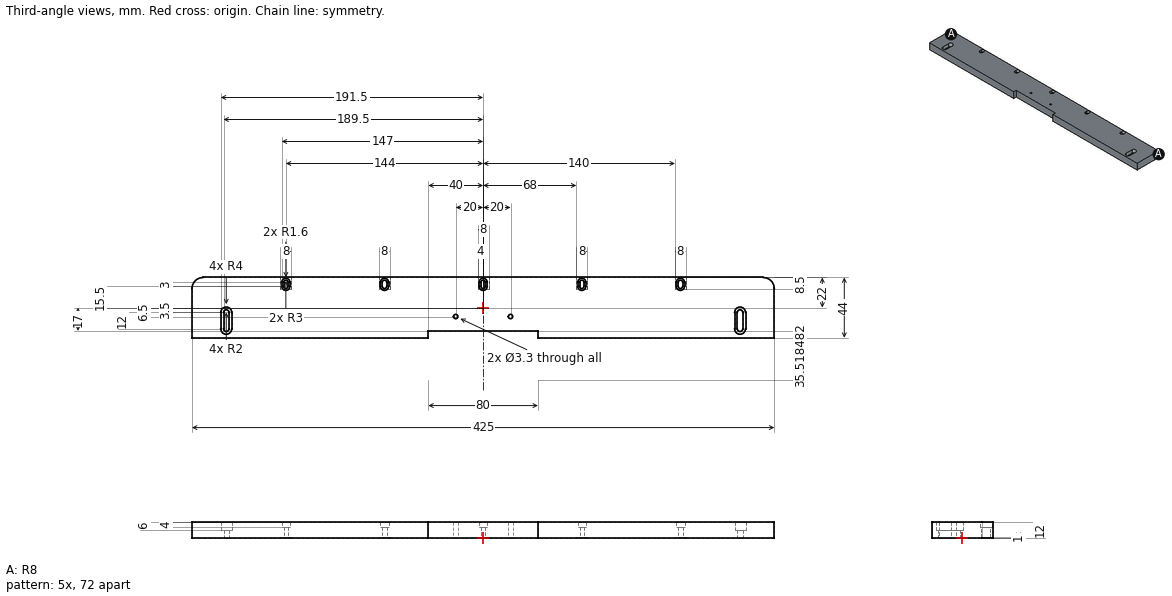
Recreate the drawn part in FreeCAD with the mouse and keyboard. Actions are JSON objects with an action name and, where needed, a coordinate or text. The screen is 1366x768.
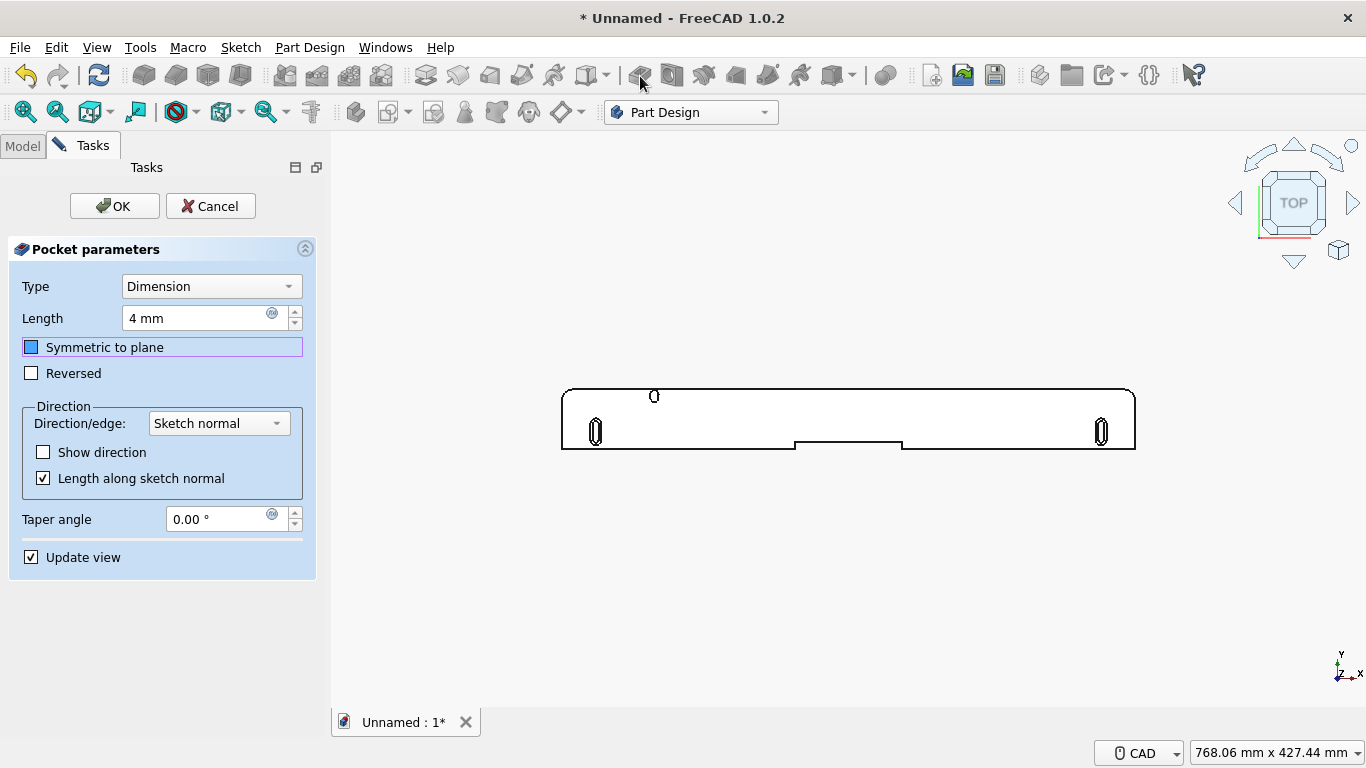
{"action": "left_click", "coordinate": [115, 206]}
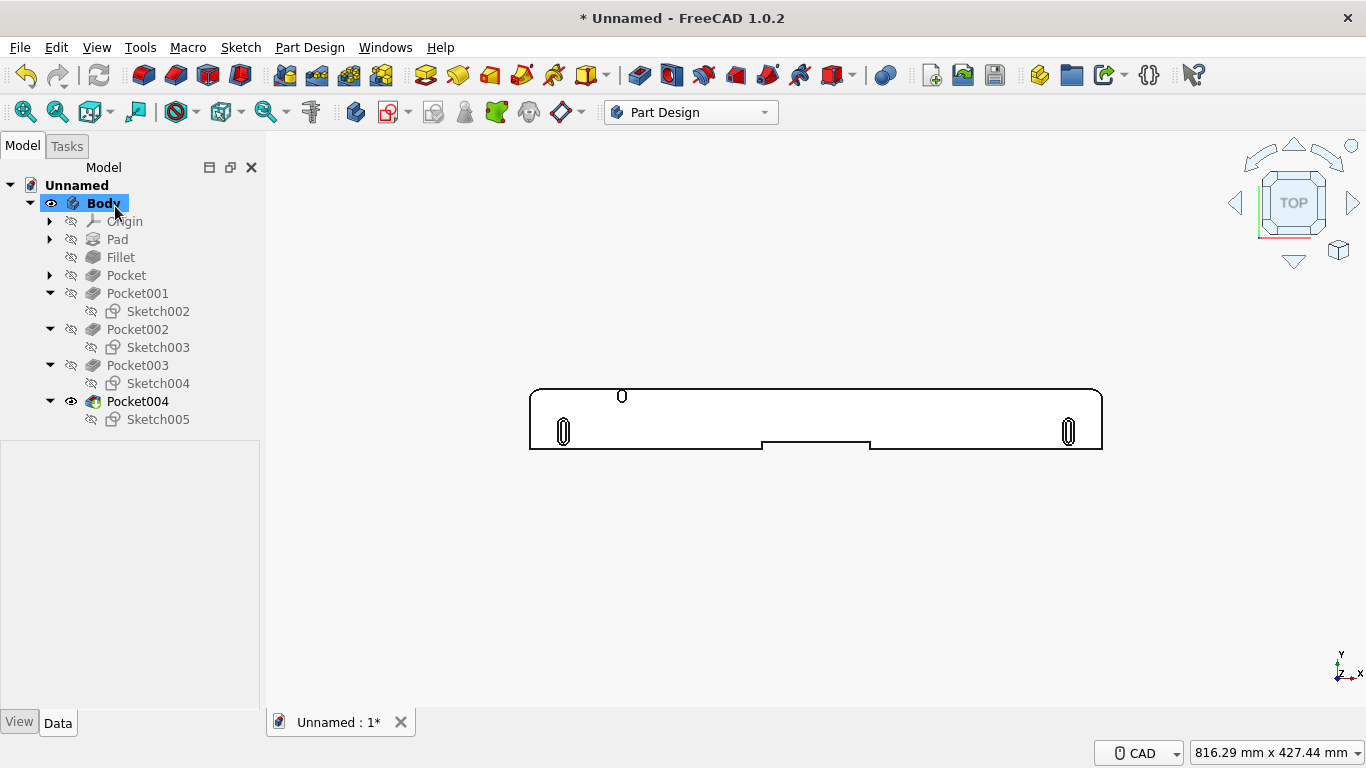
{"action": "scroll", "coordinate": [622, 393], "scroll_direction": "up", "scroll_amount": 6}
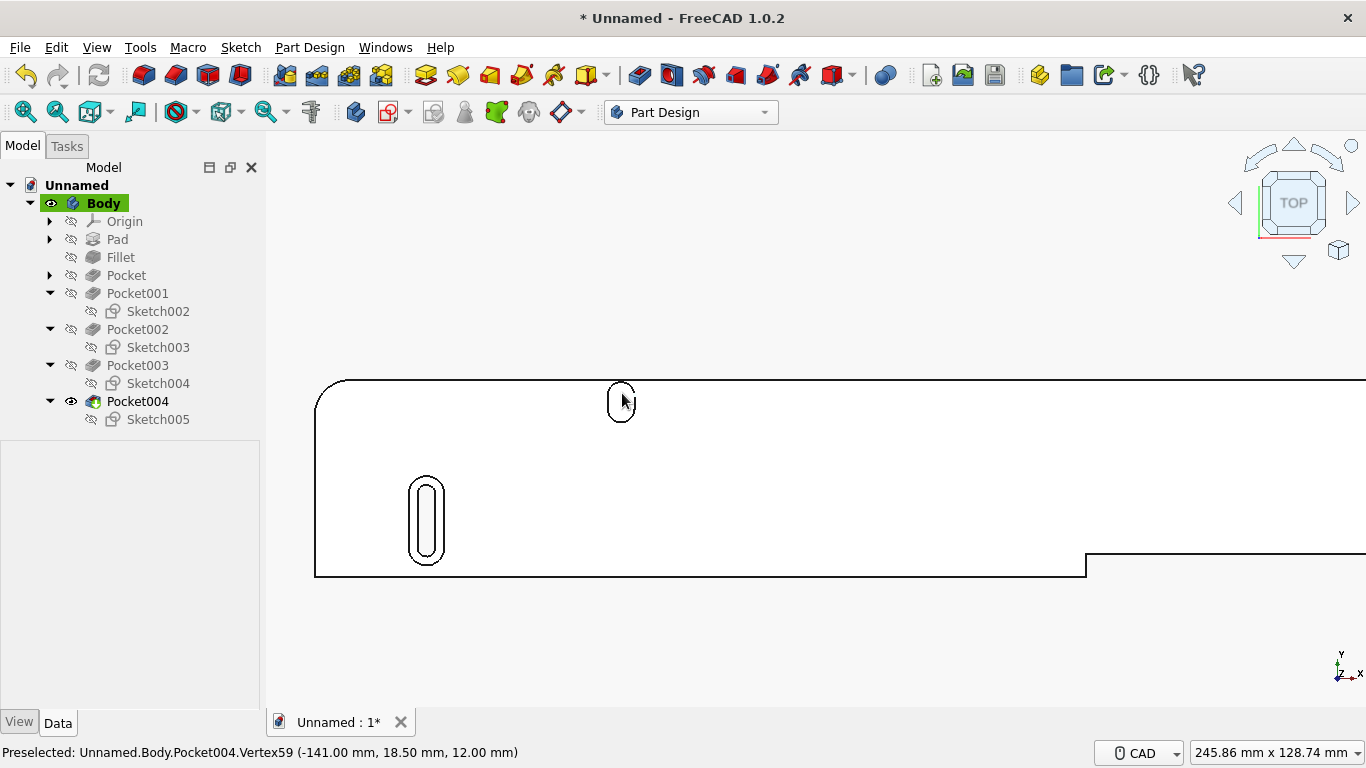
{"action": "left_click", "coordinate": [621, 395]}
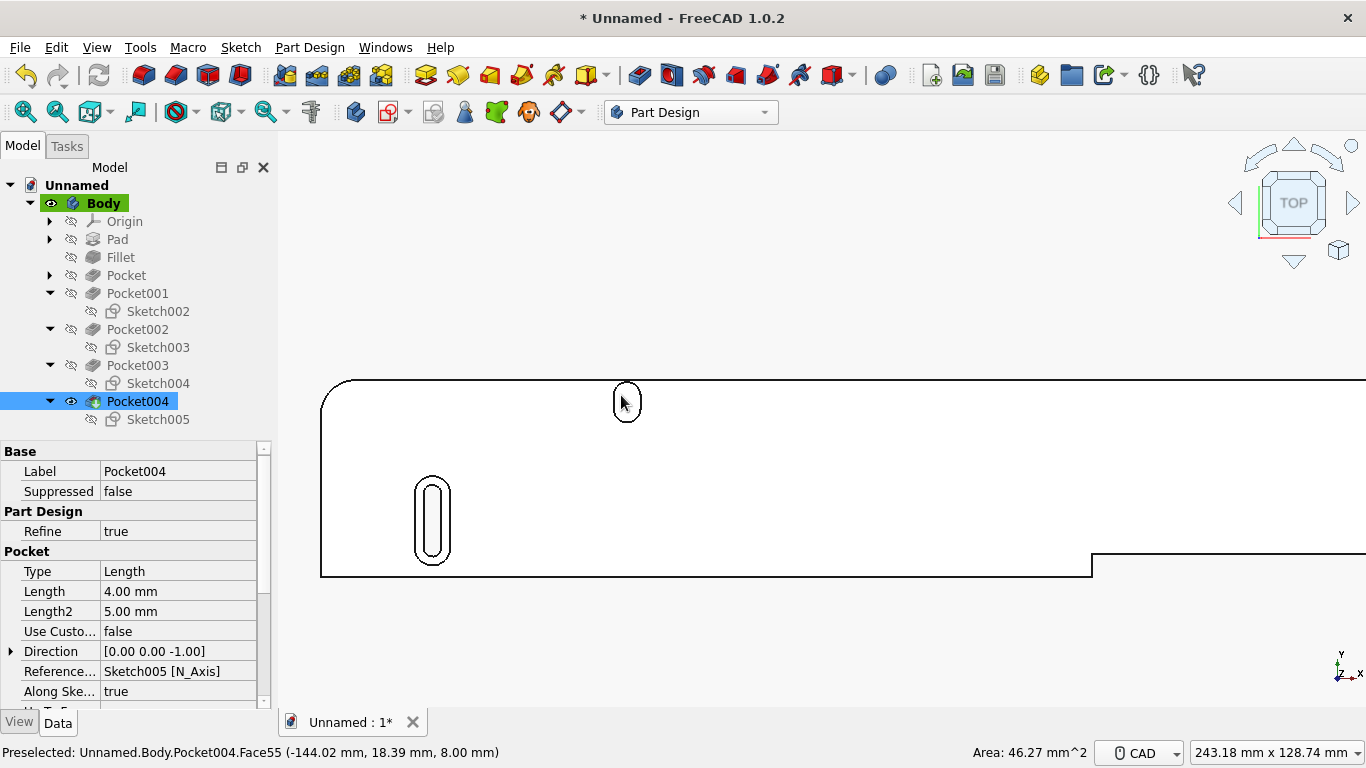
{"action": "left_click", "coordinate": [388, 112]}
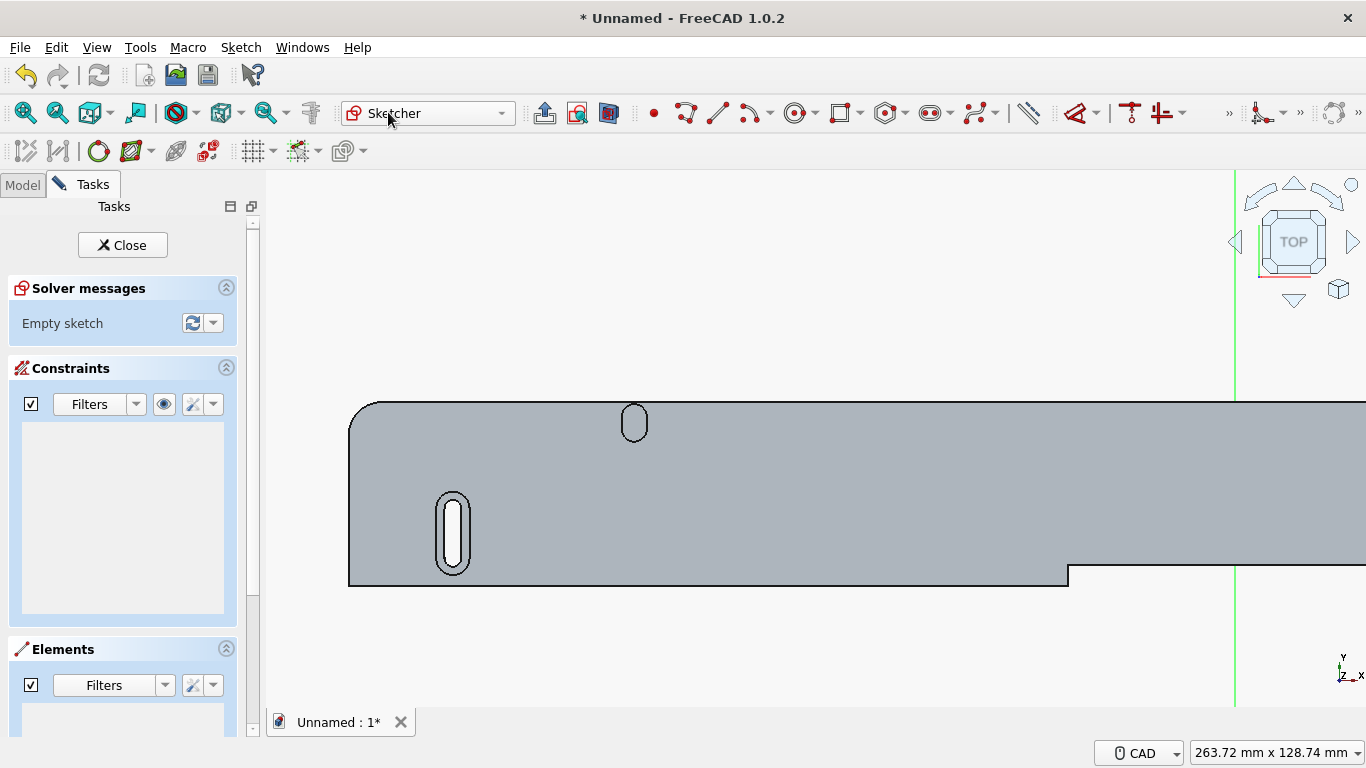
{"action": "scroll", "coordinate": [625, 422], "scroll_direction": "up", "scroll_amount": 13}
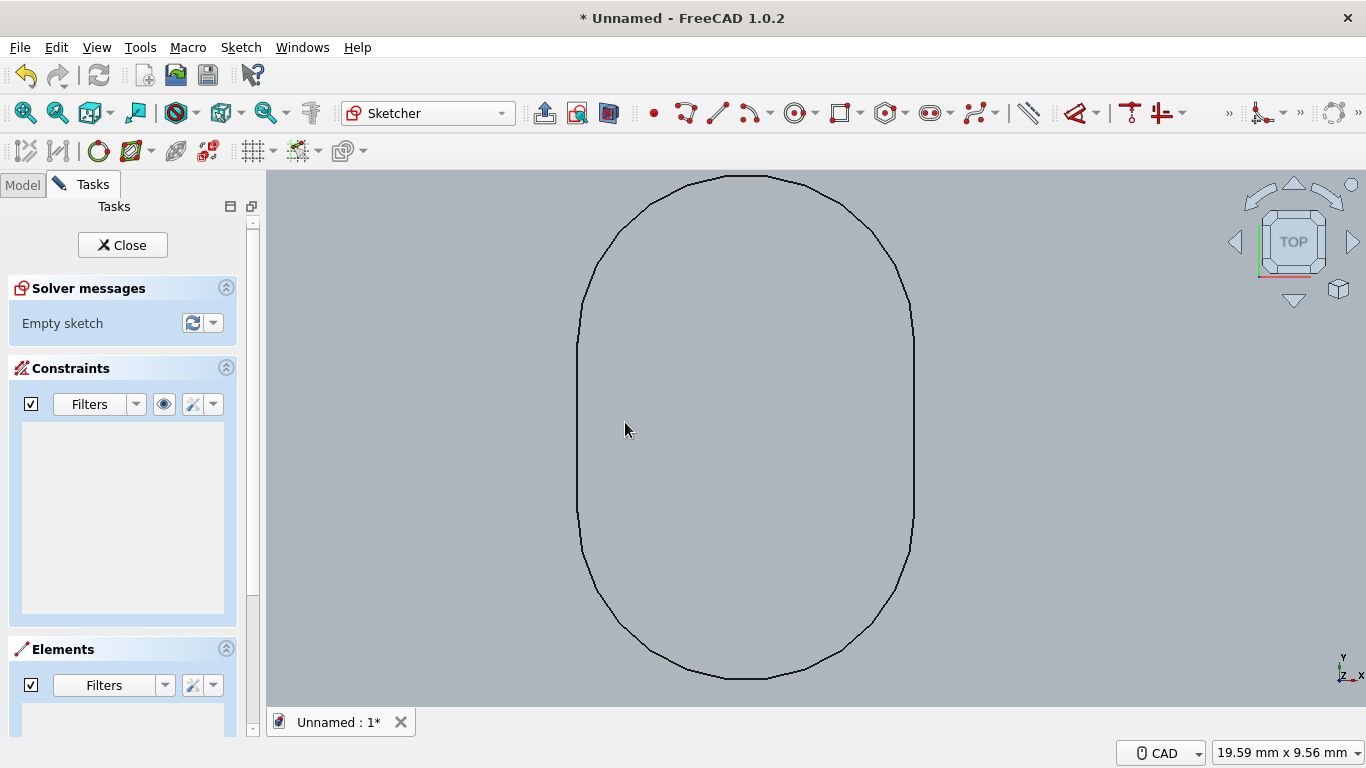
{"action": "left_click", "coordinate": [930, 114]}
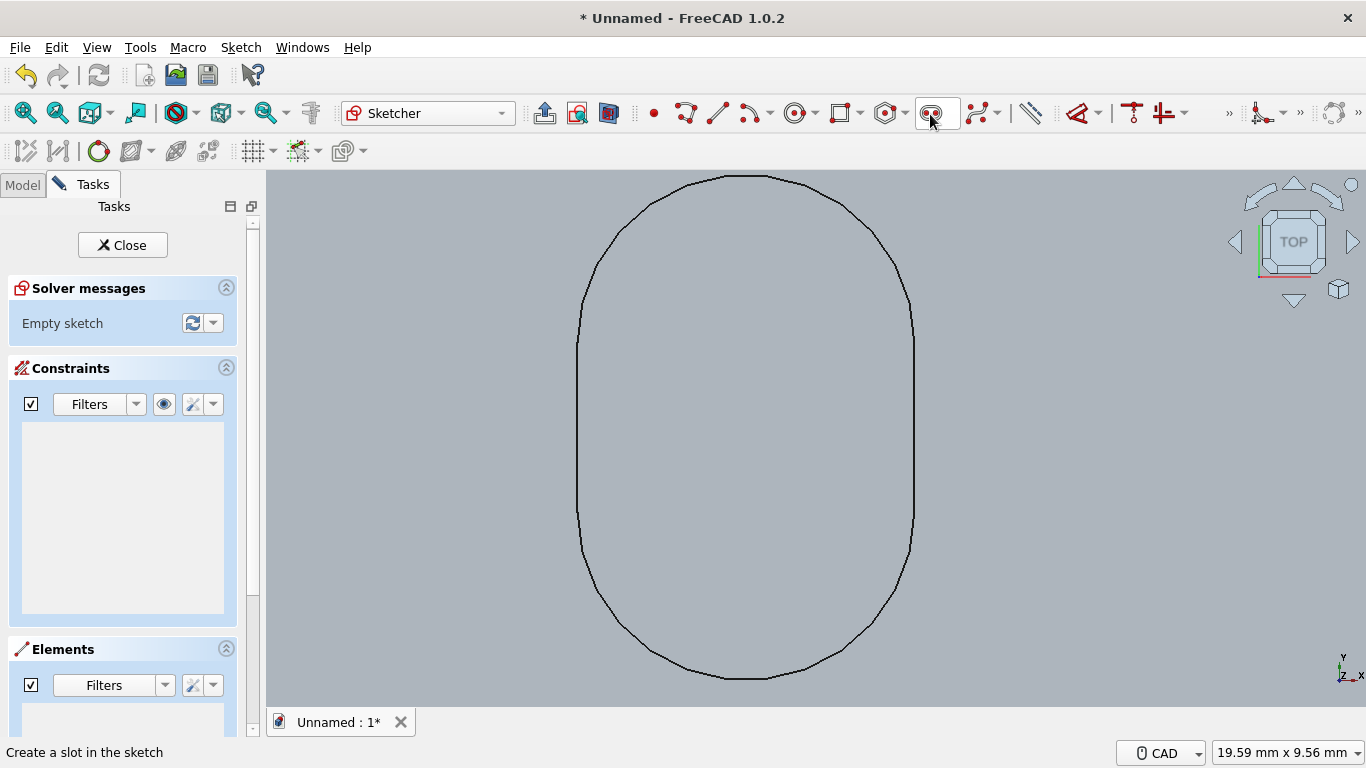
{"action": "left_click", "coordinate": [746, 512]}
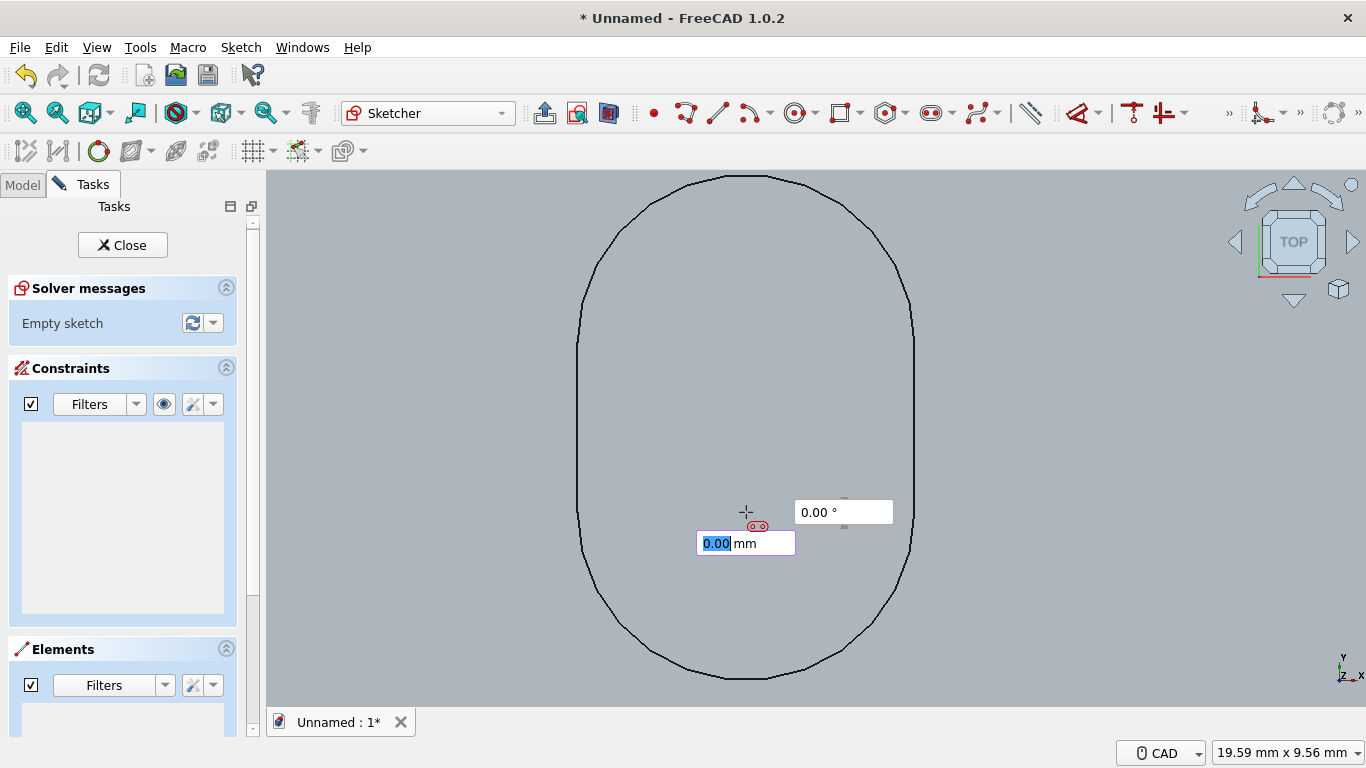
{"action": "left_click", "coordinate": [746, 343]}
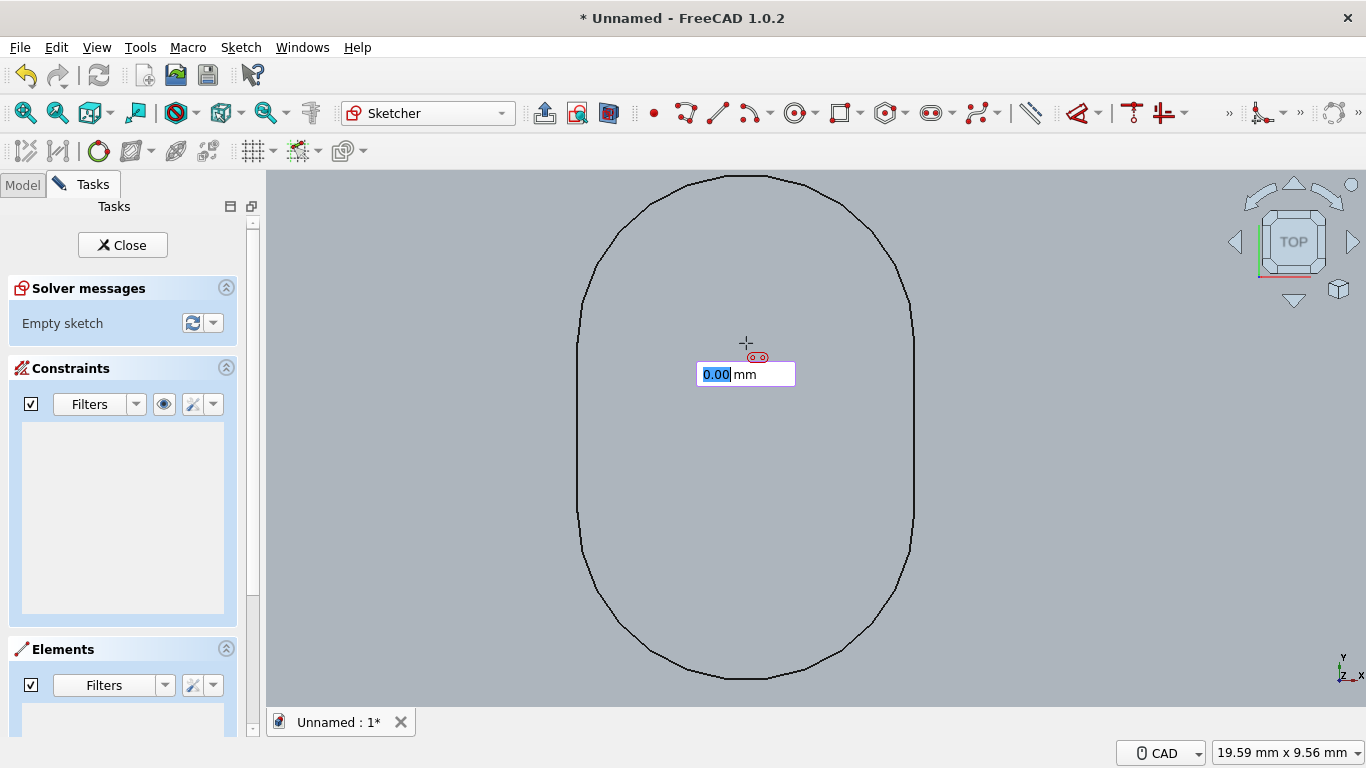
{"action": "left_click", "coordinate": [836, 428]}
{"action": "key", "text": "Escape"}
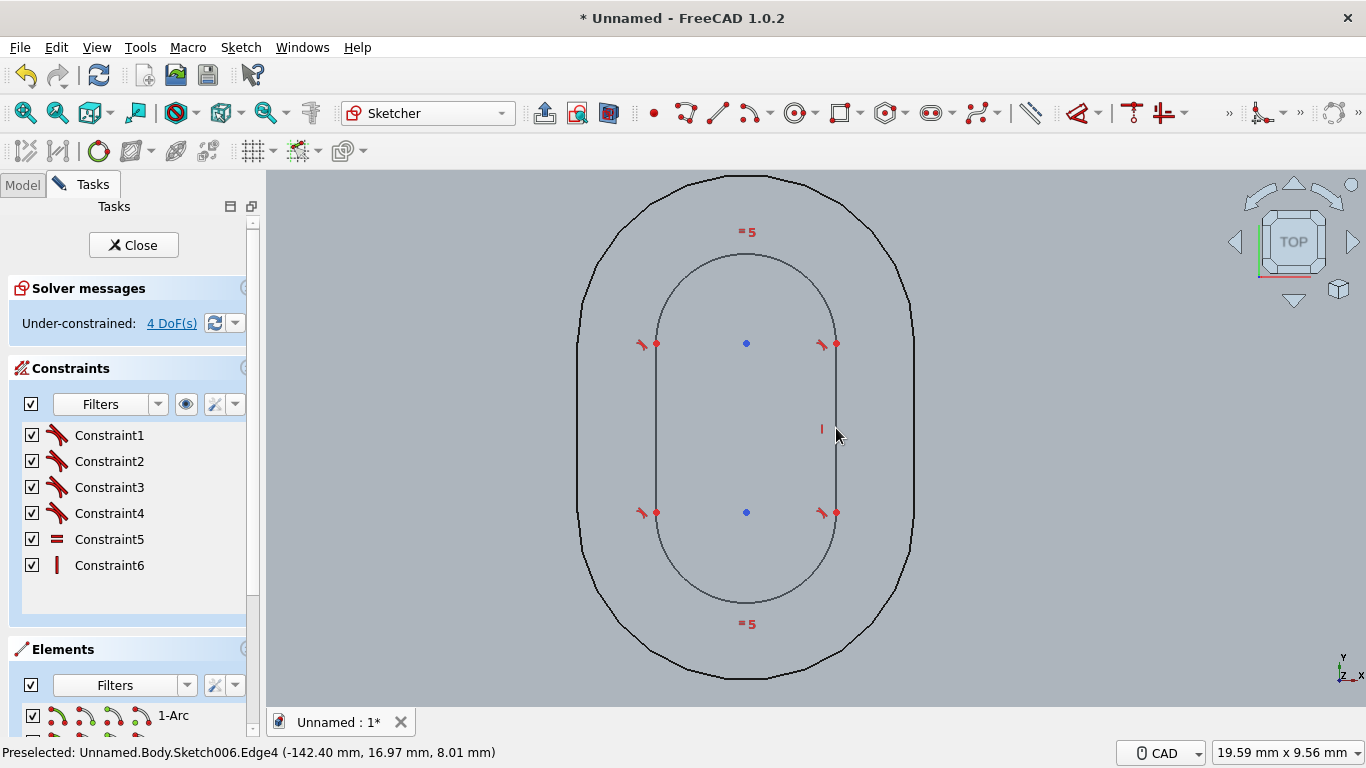
{"action": "left_click", "coordinate": [1078, 114]}